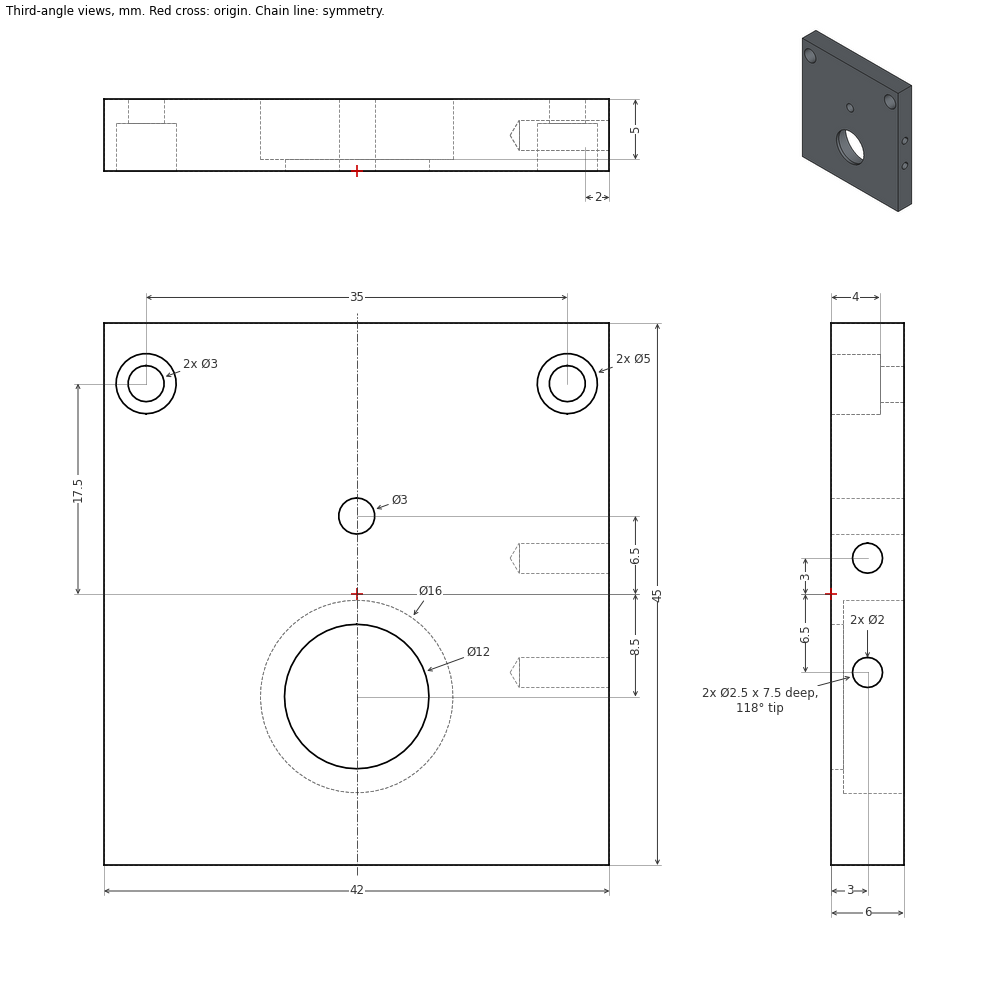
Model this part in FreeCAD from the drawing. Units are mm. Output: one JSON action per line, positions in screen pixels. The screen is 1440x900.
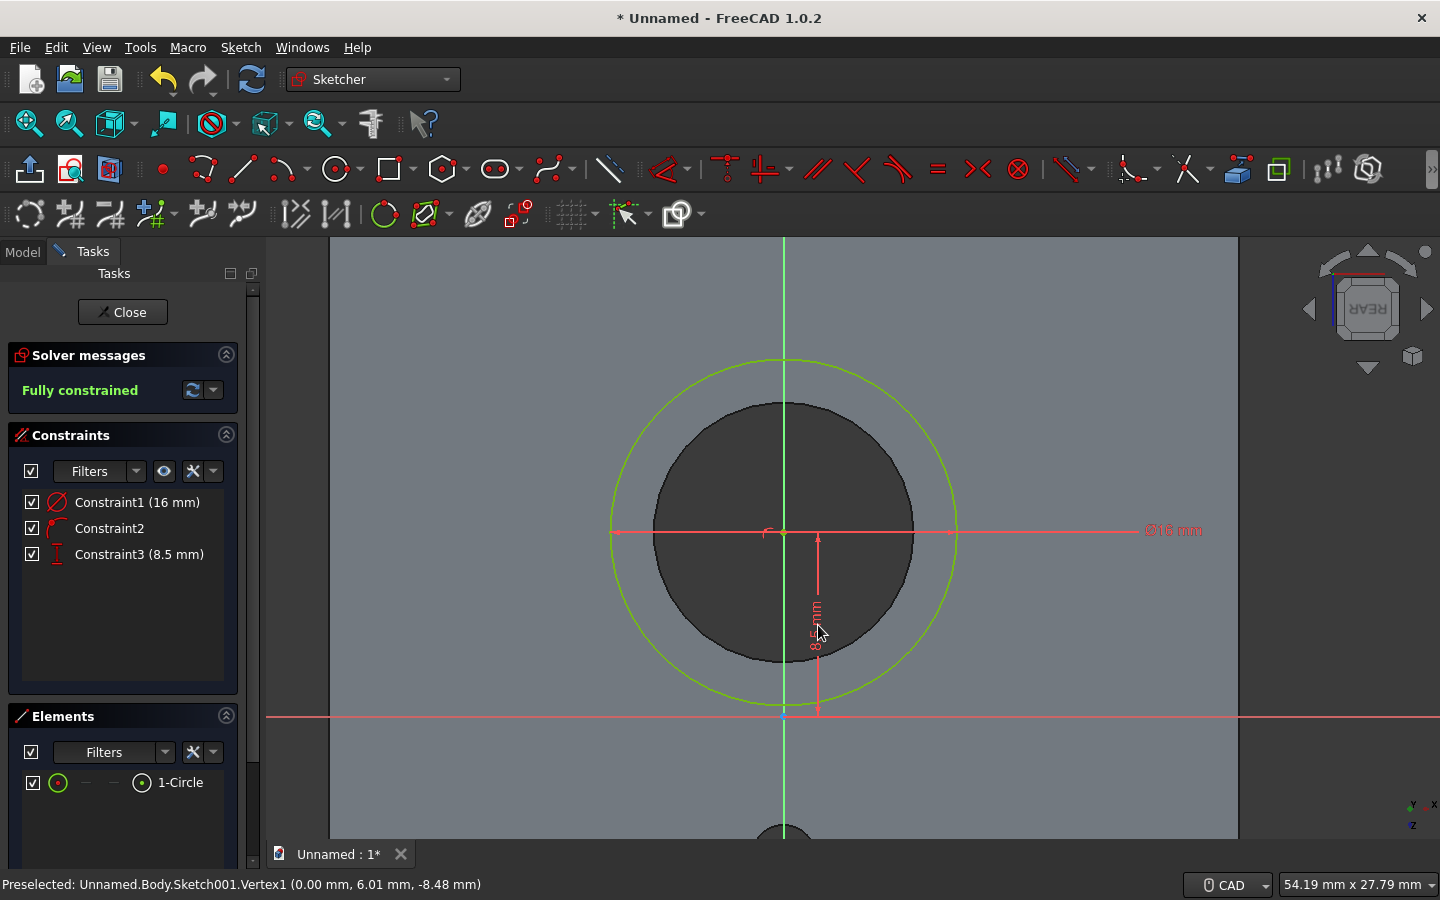
{"action": "left_click", "coordinate": [123, 312]}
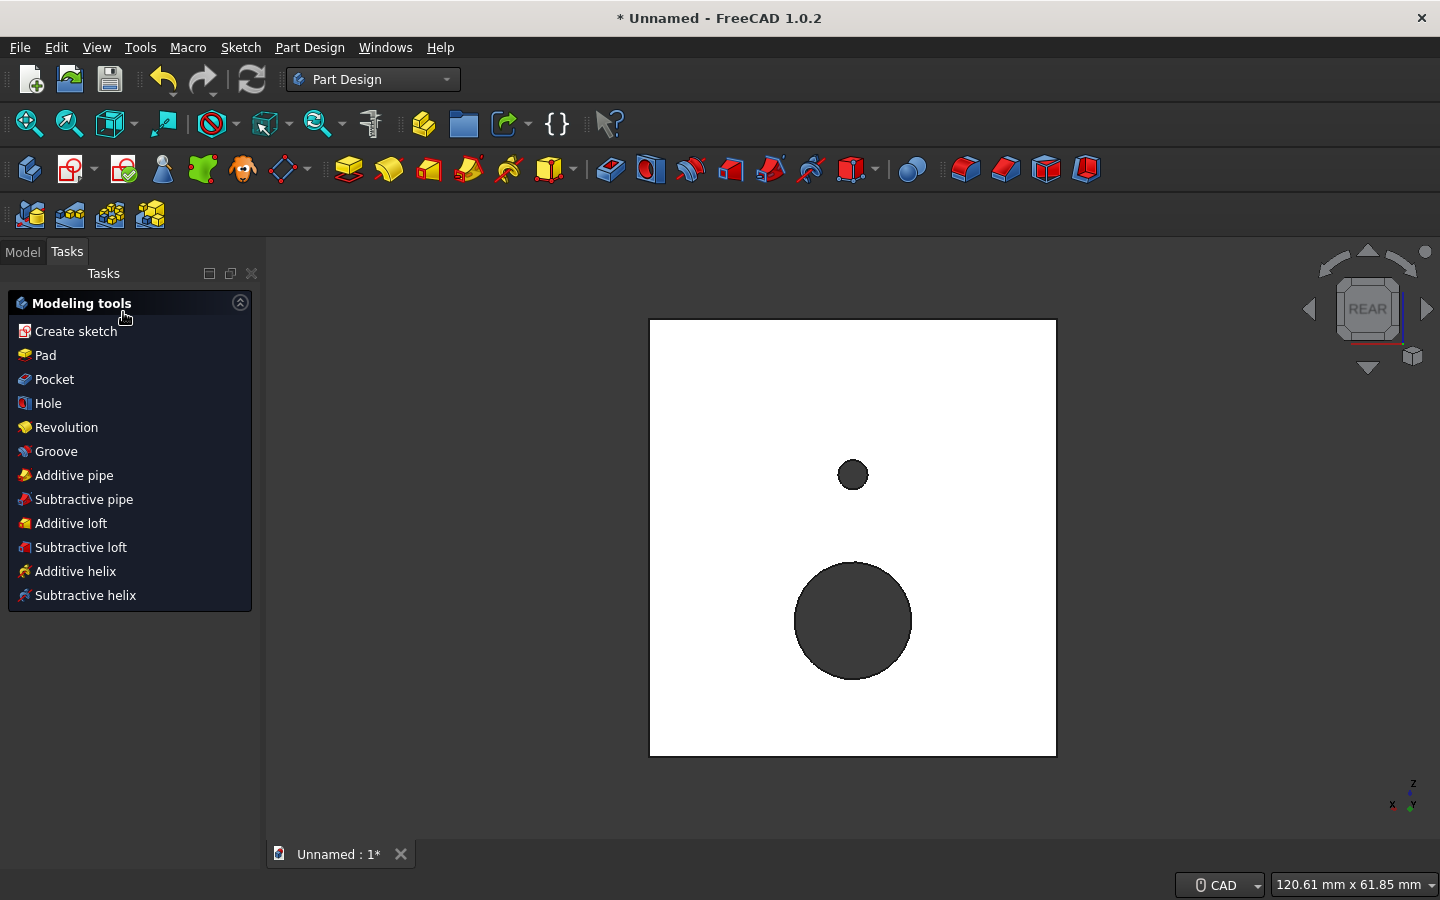
{"action": "left_click", "coordinate": [612, 170]}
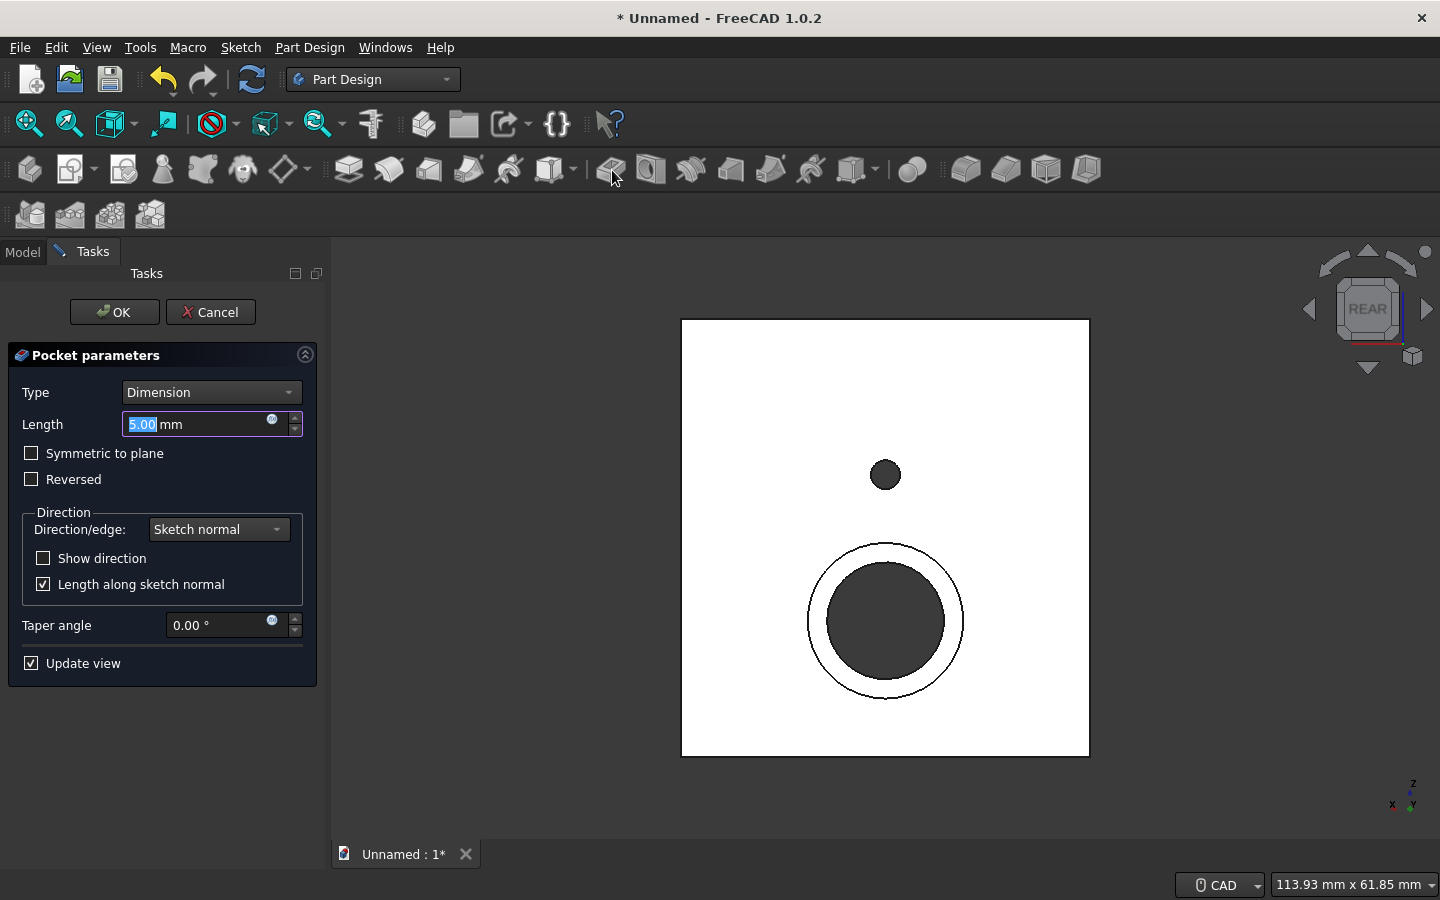
{"action": "type", "text": "5"}
{"action": "key", "text": "Tab"}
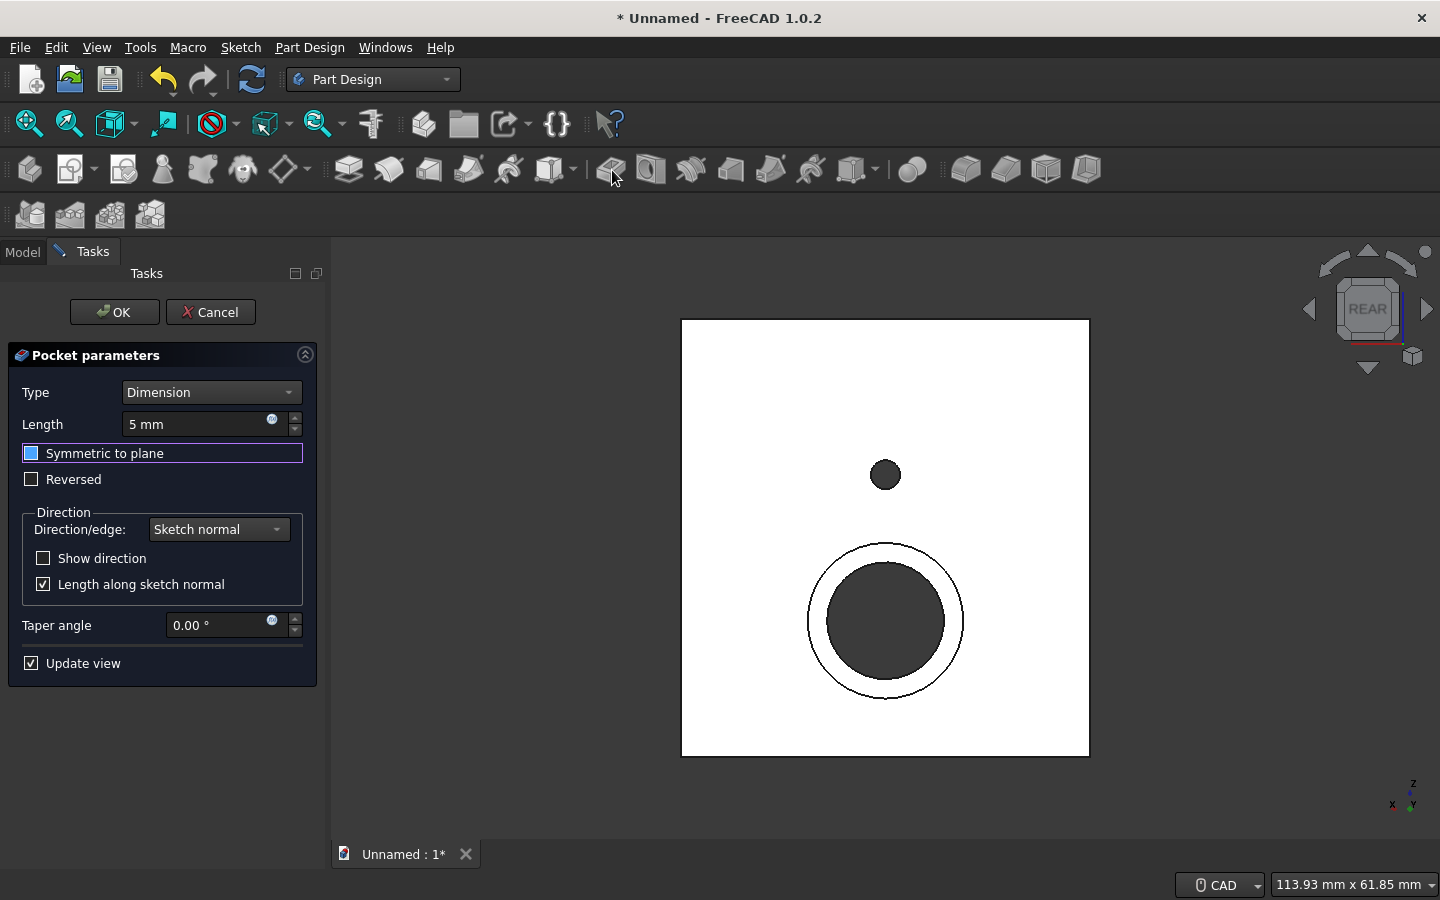
{"action": "left_click", "coordinate": [115, 312]}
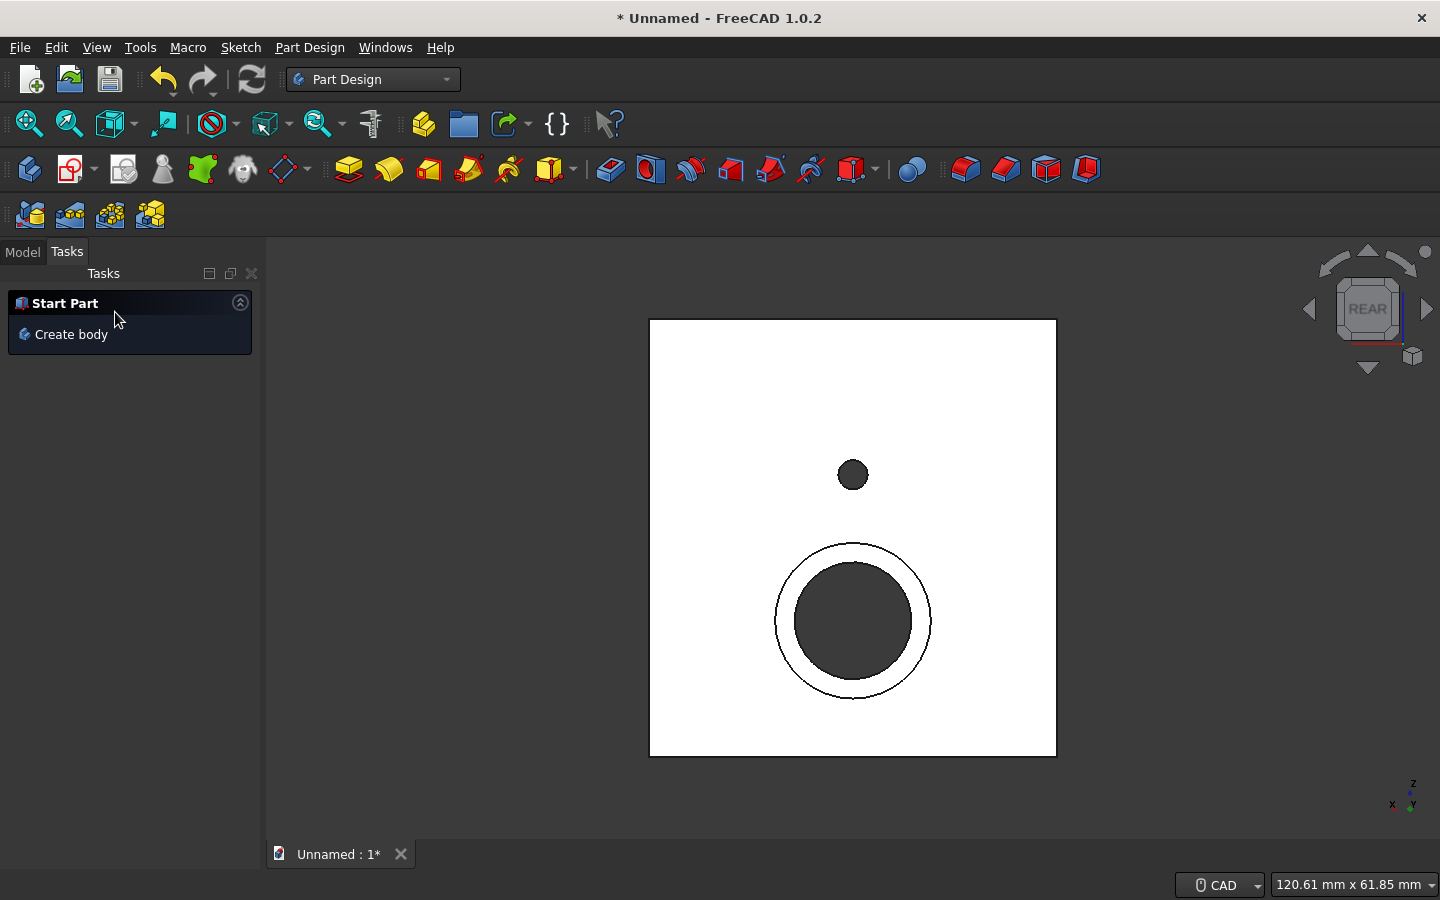
{"action": "left_click", "coordinate": [736, 412]}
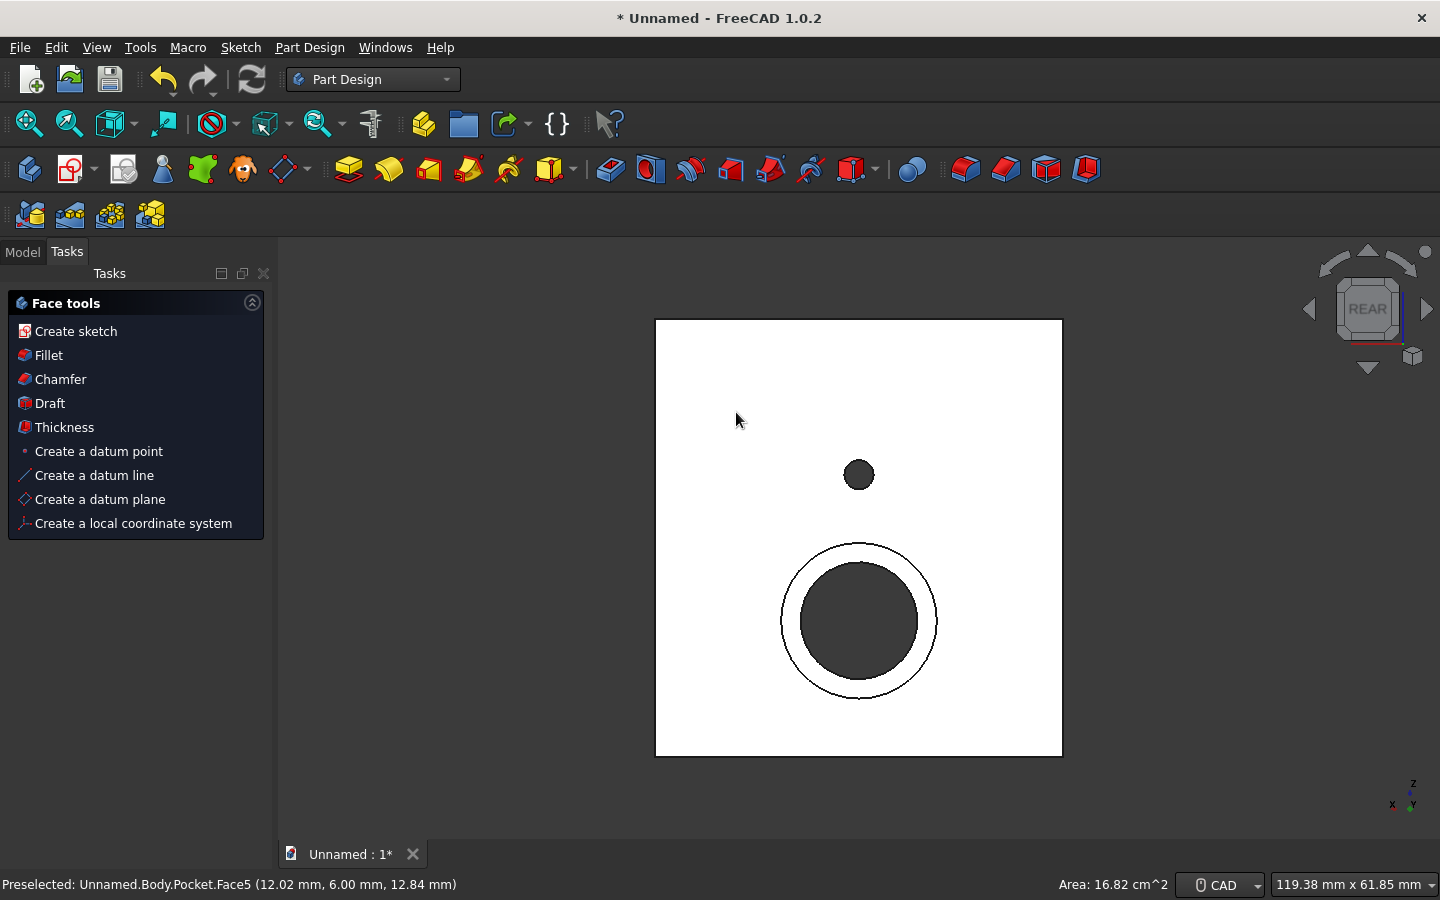
{"action": "left_click", "coordinate": [70, 170]}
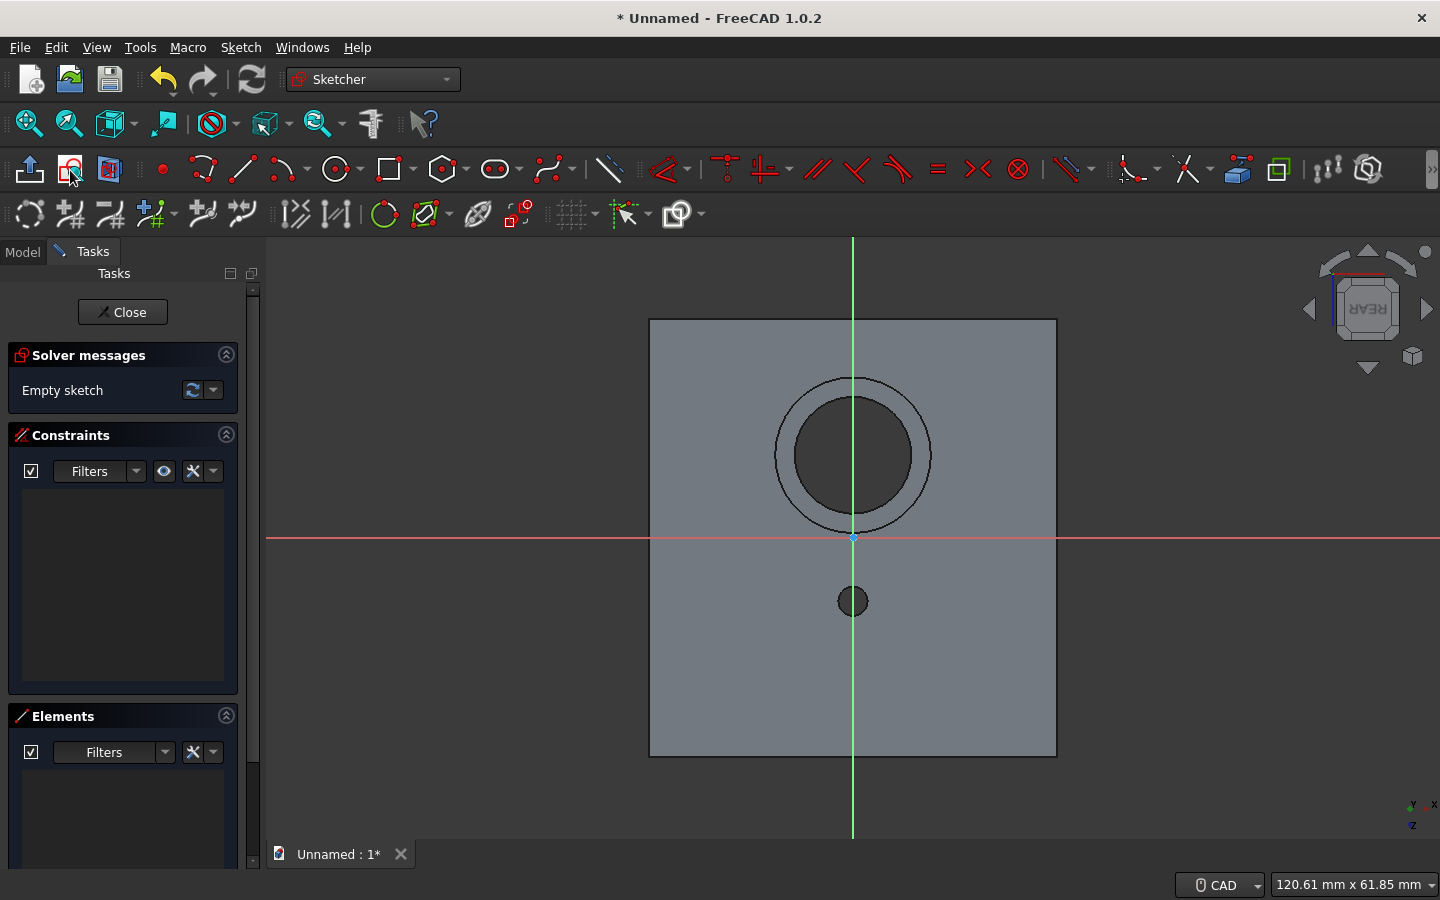
{"action": "scroll", "coordinate": [936, 743], "scroll_direction": "up", "scroll_amount": 3}